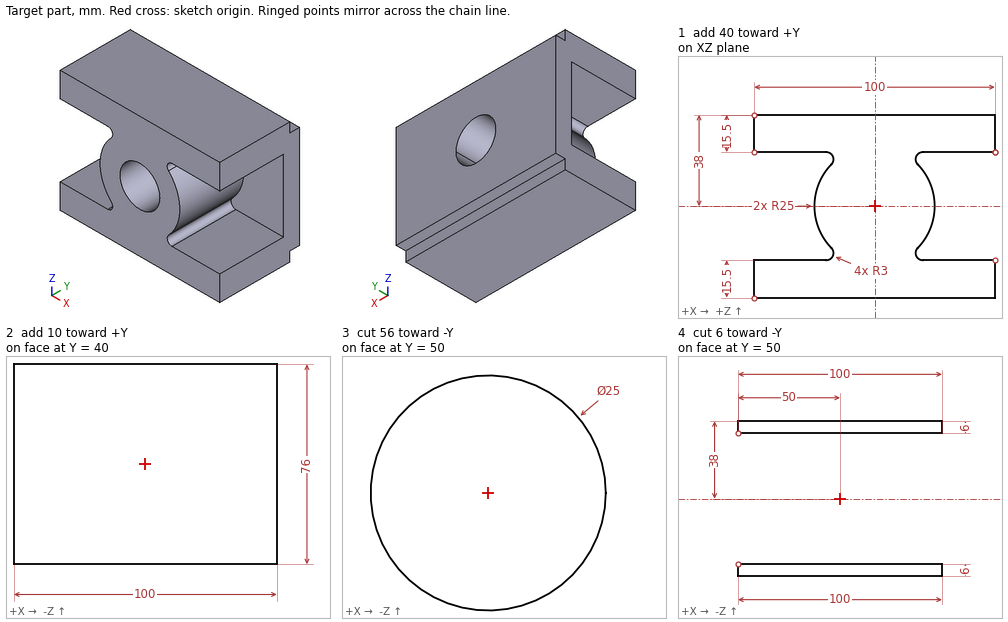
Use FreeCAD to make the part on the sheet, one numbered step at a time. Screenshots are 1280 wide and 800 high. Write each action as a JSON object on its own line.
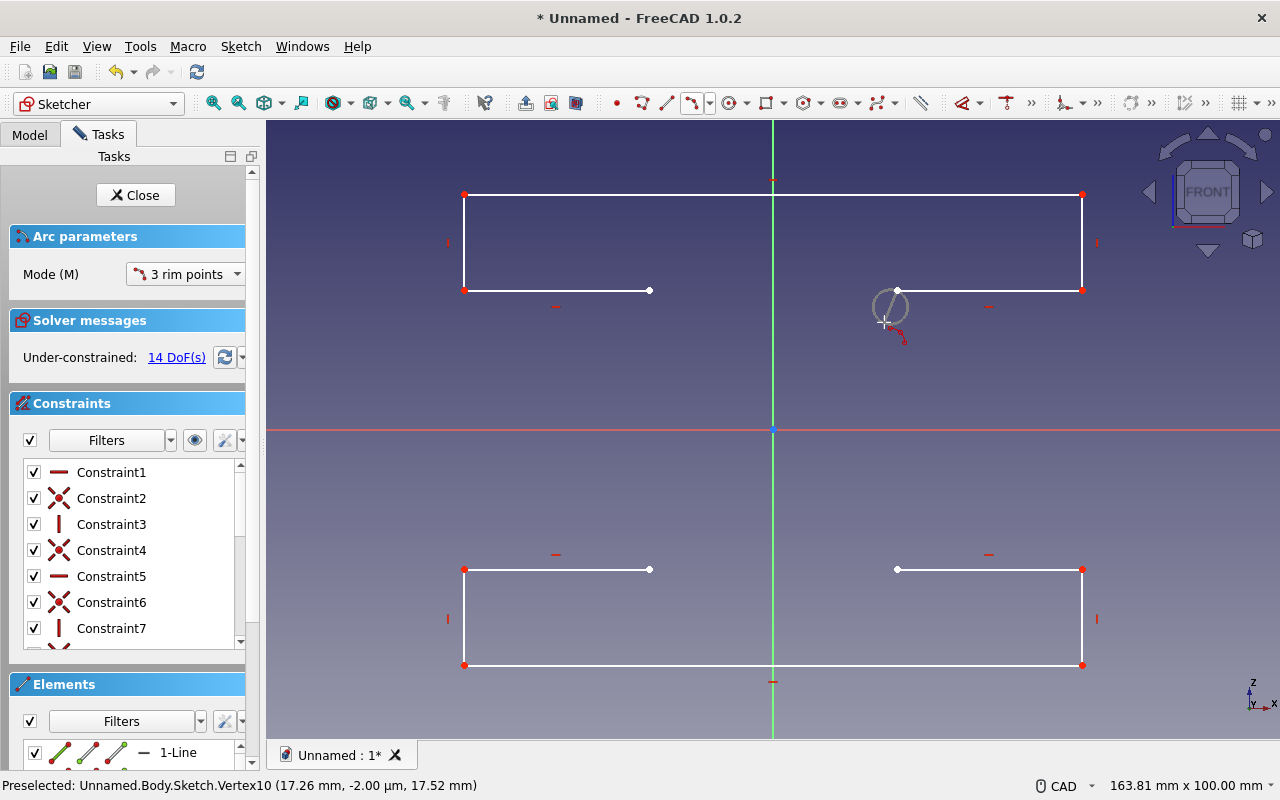
{"action": "scroll", "coordinate": [880, 302], "scroll_direction": "up", "scroll_amount": 2}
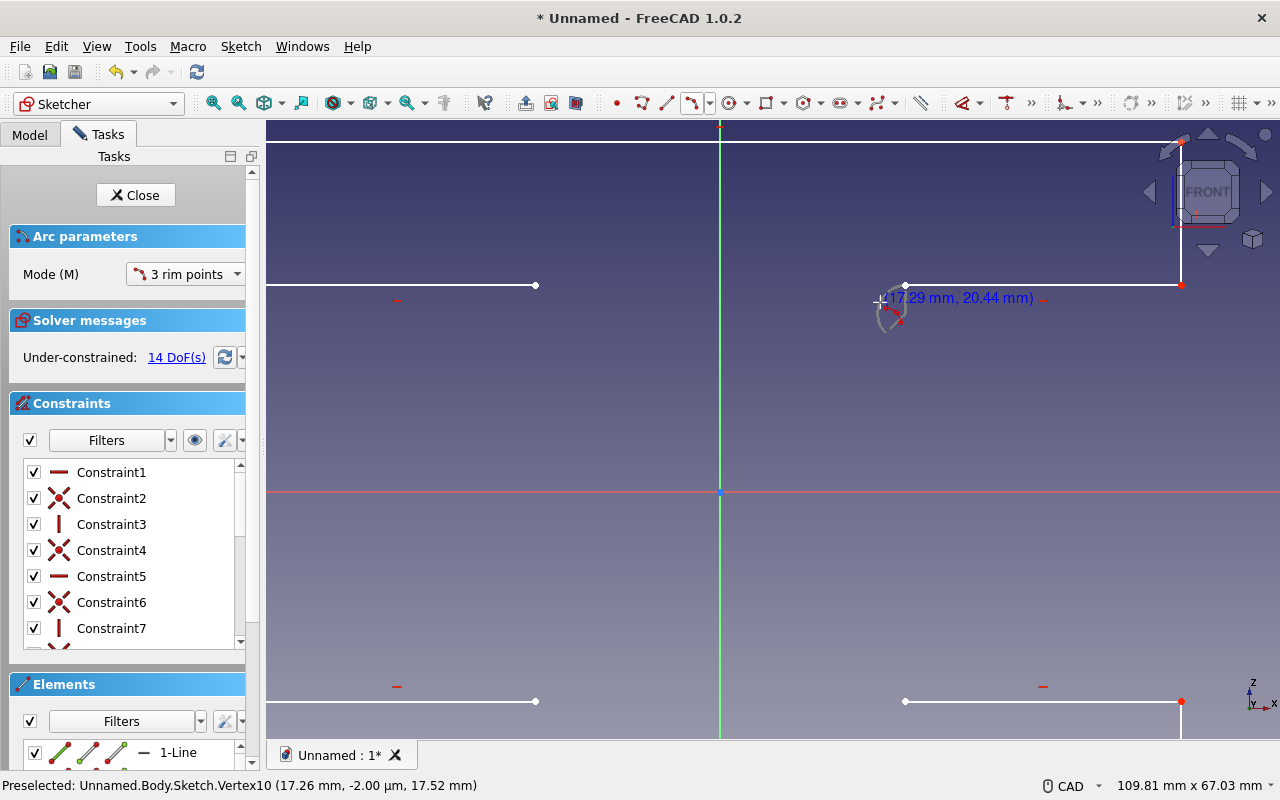
{"action": "left_click", "coordinate": [880, 301]}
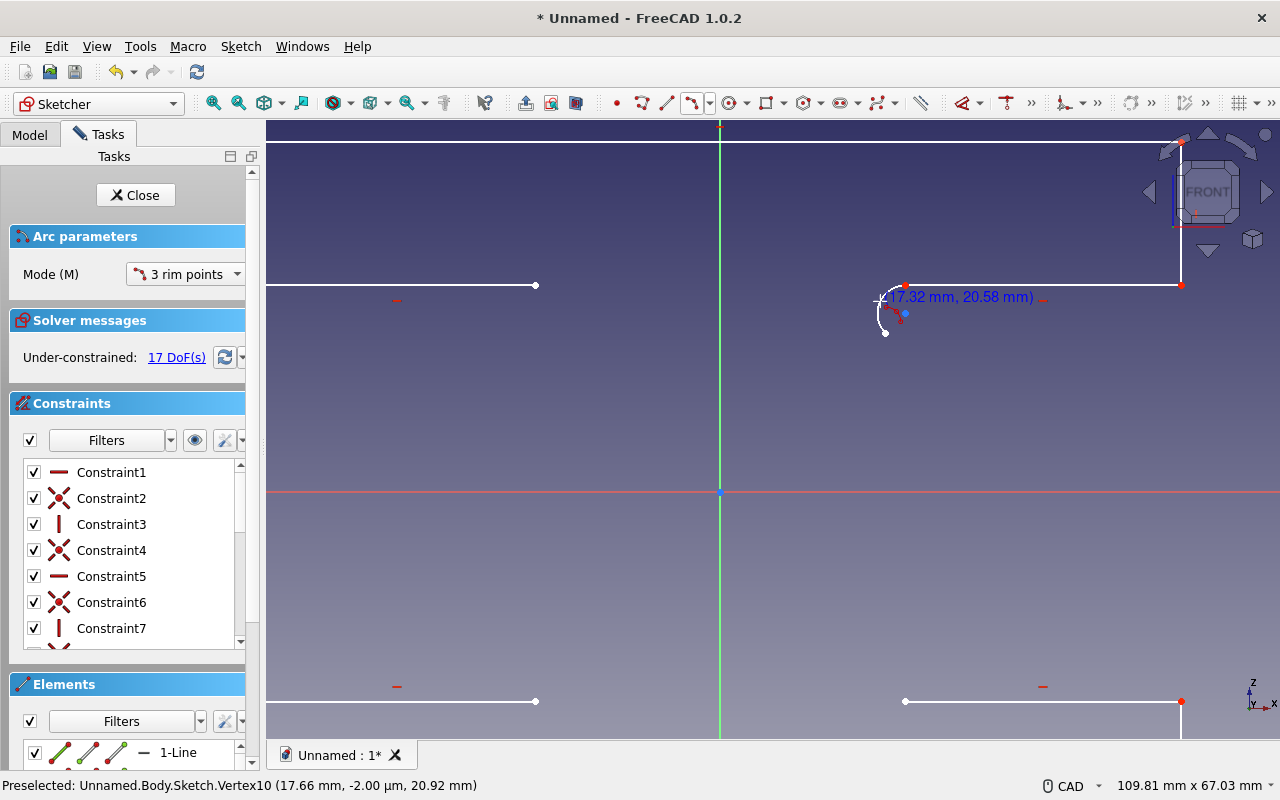
{"action": "left_click", "coordinate": [886, 333]}
{"action": "left_click", "coordinate": [886, 653]}
{"action": "left_click", "coordinate": [948, 527]}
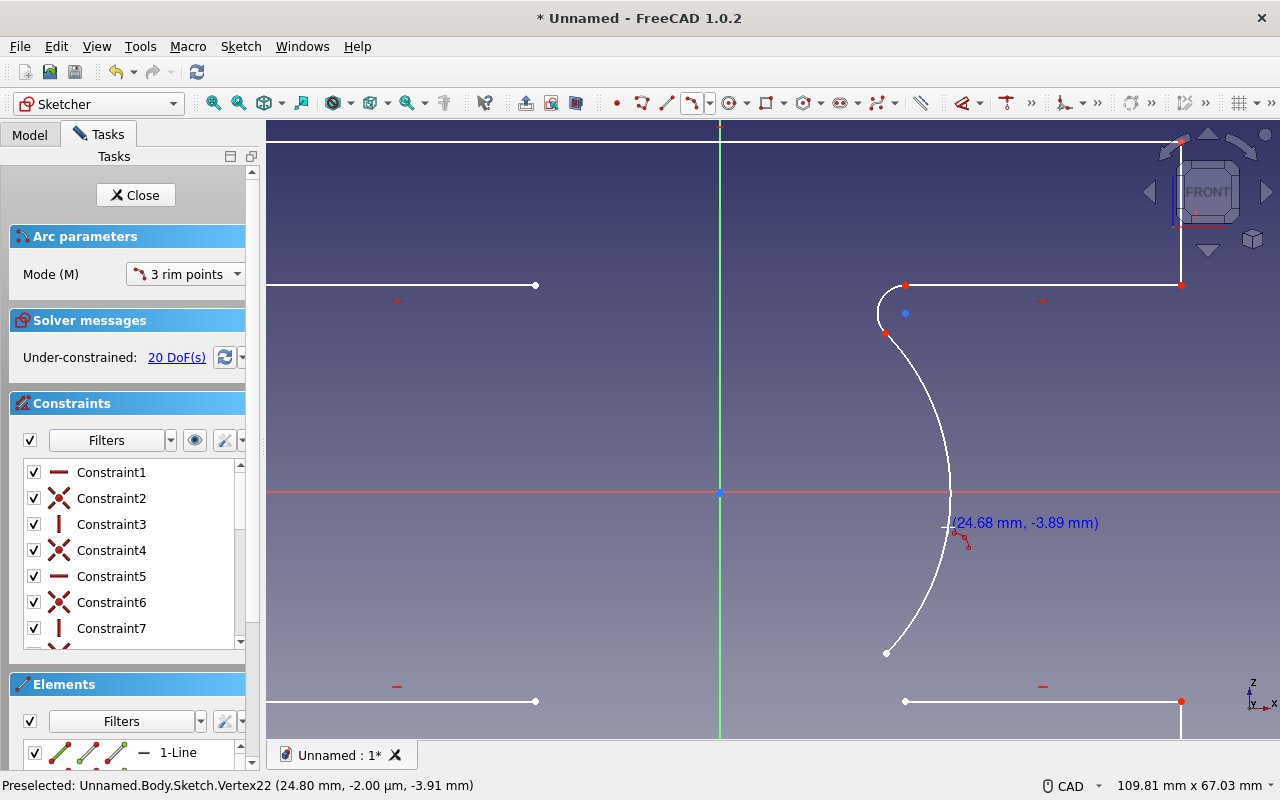
{"action": "left_click", "coordinate": [886, 654]}
{"action": "left_click", "coordinate": [905, 702]}
{"action": "left_click", "coordinate": [880, 683]}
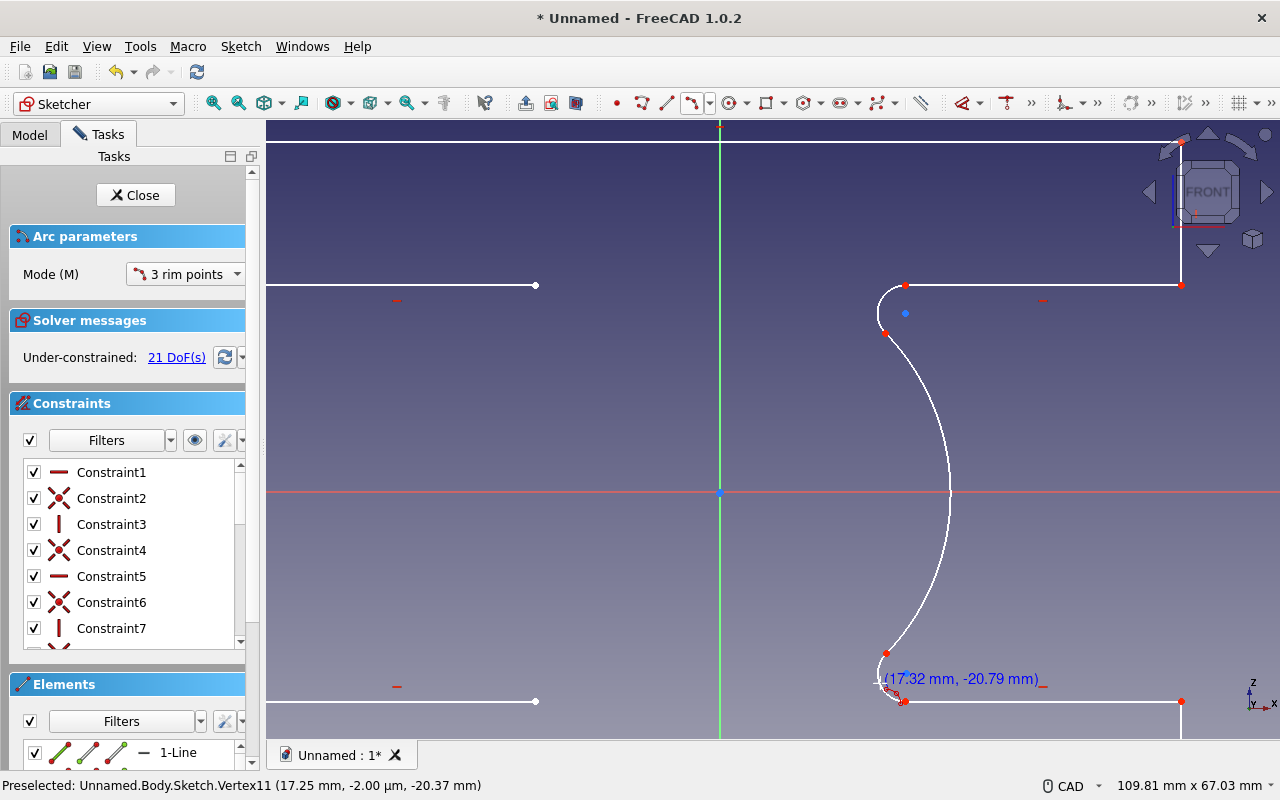
{"action": "left_click", "coordinate": [535, 702]}
{"action": "left_click", "coordinate": [554, 653]}
{"action": "left_click", "coordinate": [560, 683]}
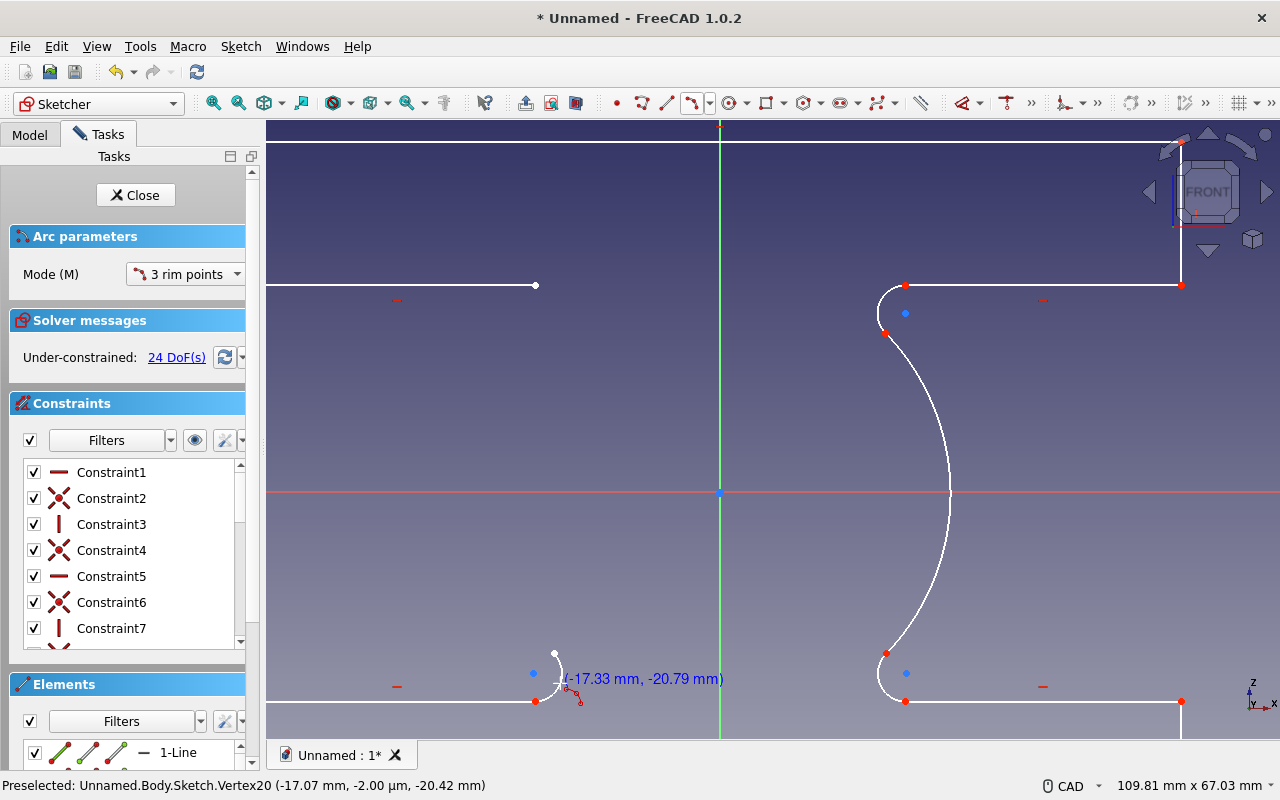
{"action": "left_click", "coordinate": [554, 654]}
{"action": "left_click", "coordinate": [554, 331]}
{"action": "left_click", "coordinate": [492, 457]}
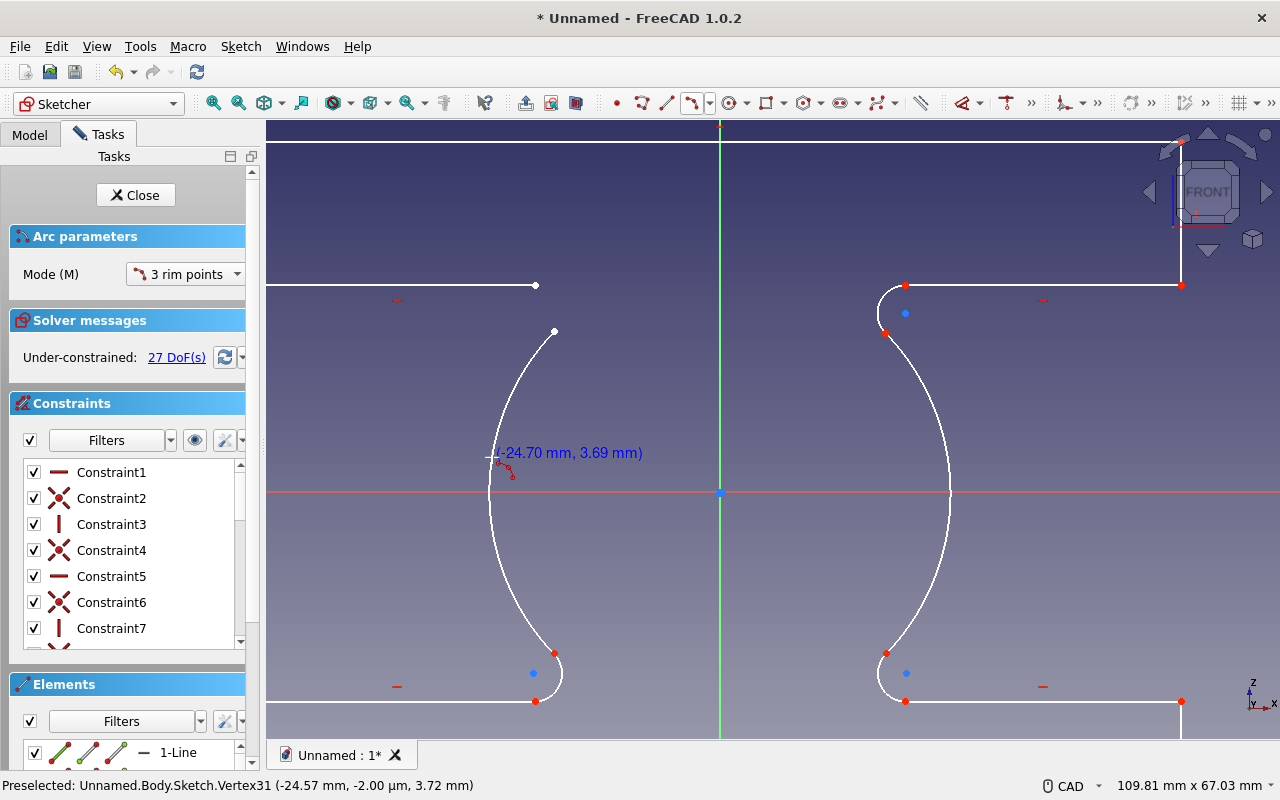
{"action": "left_click", "coordinate": [554, 332]}
{"action": "left_click", "coordinate": [535, 285]}
{"action": "left_click", "coordinate": [560, 301]}
{"action": "key", "text": "Escape"}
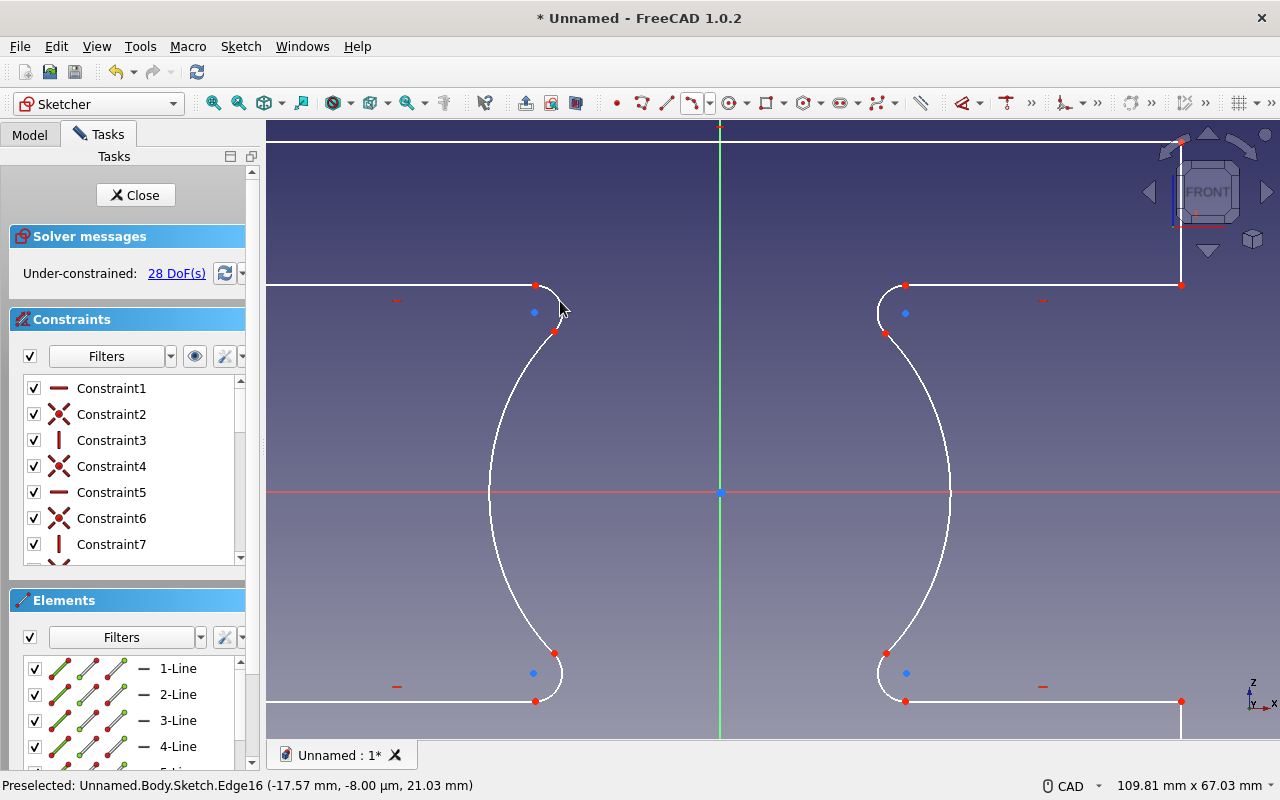
{"action": "left_click", "coordinate": [452, 285]}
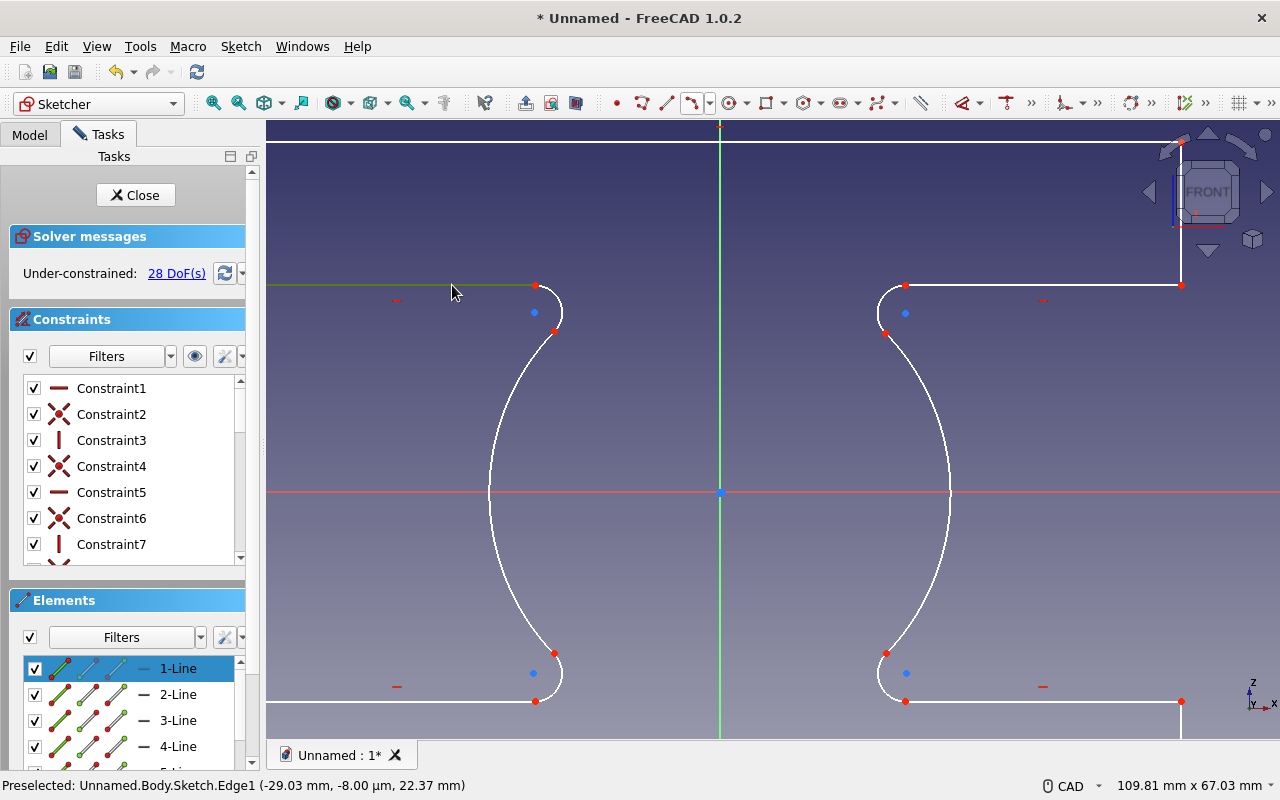
{"action": "left_click", "coordinate": [562, 315]}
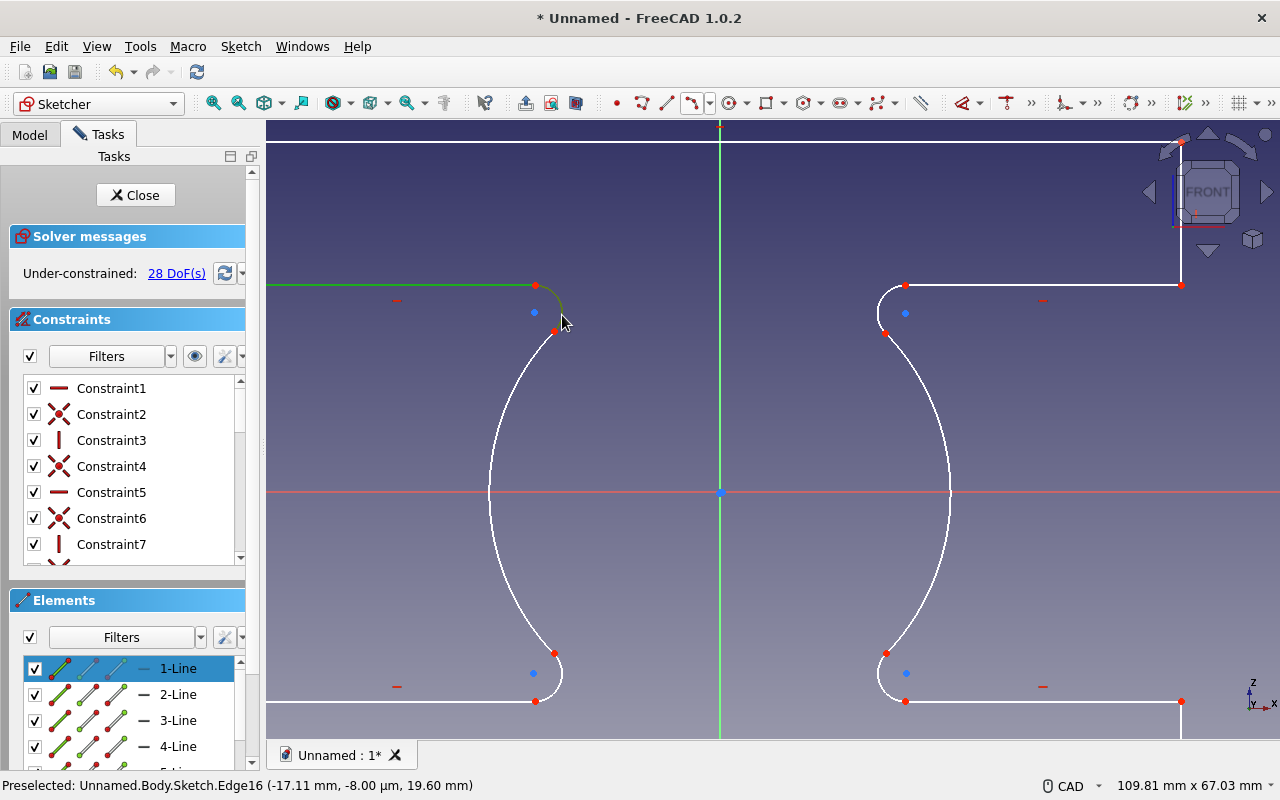
{"action": "key", "text": "t"}